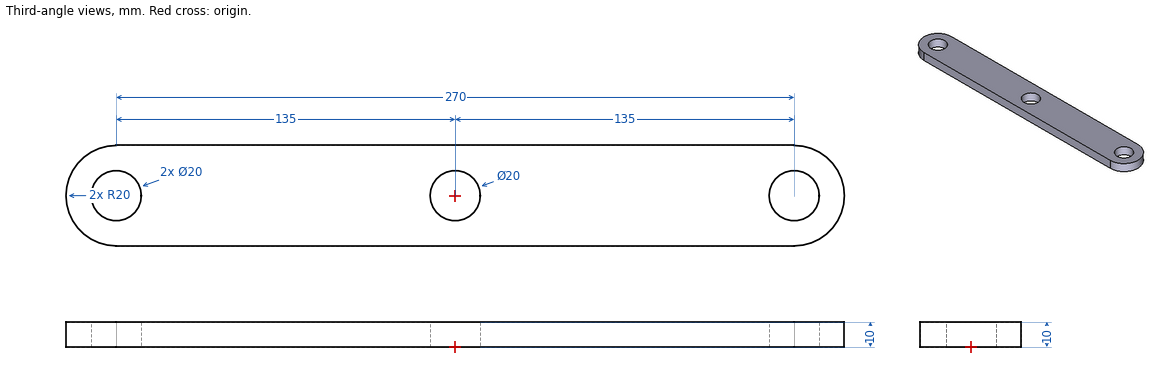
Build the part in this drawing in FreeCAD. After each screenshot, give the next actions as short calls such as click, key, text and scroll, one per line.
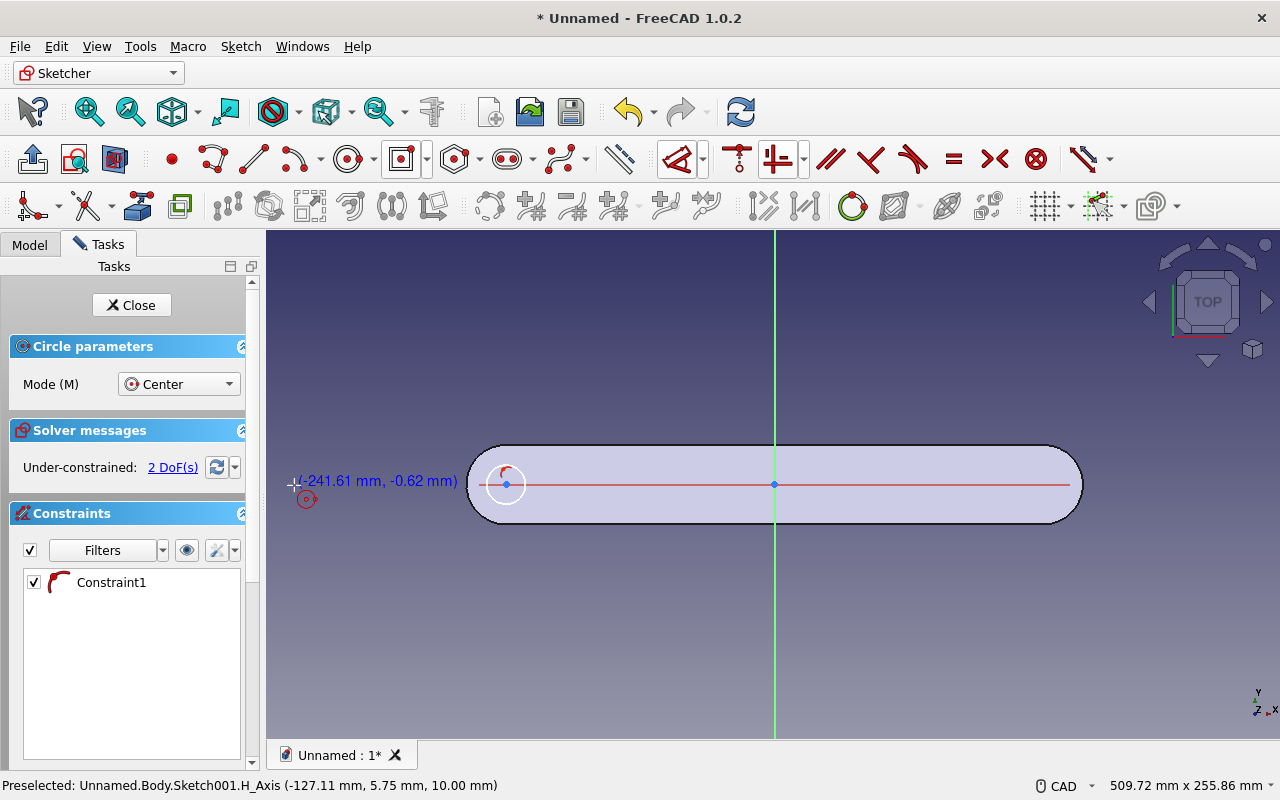
click(1043, 485)
click(1057, 471)
key(Escape)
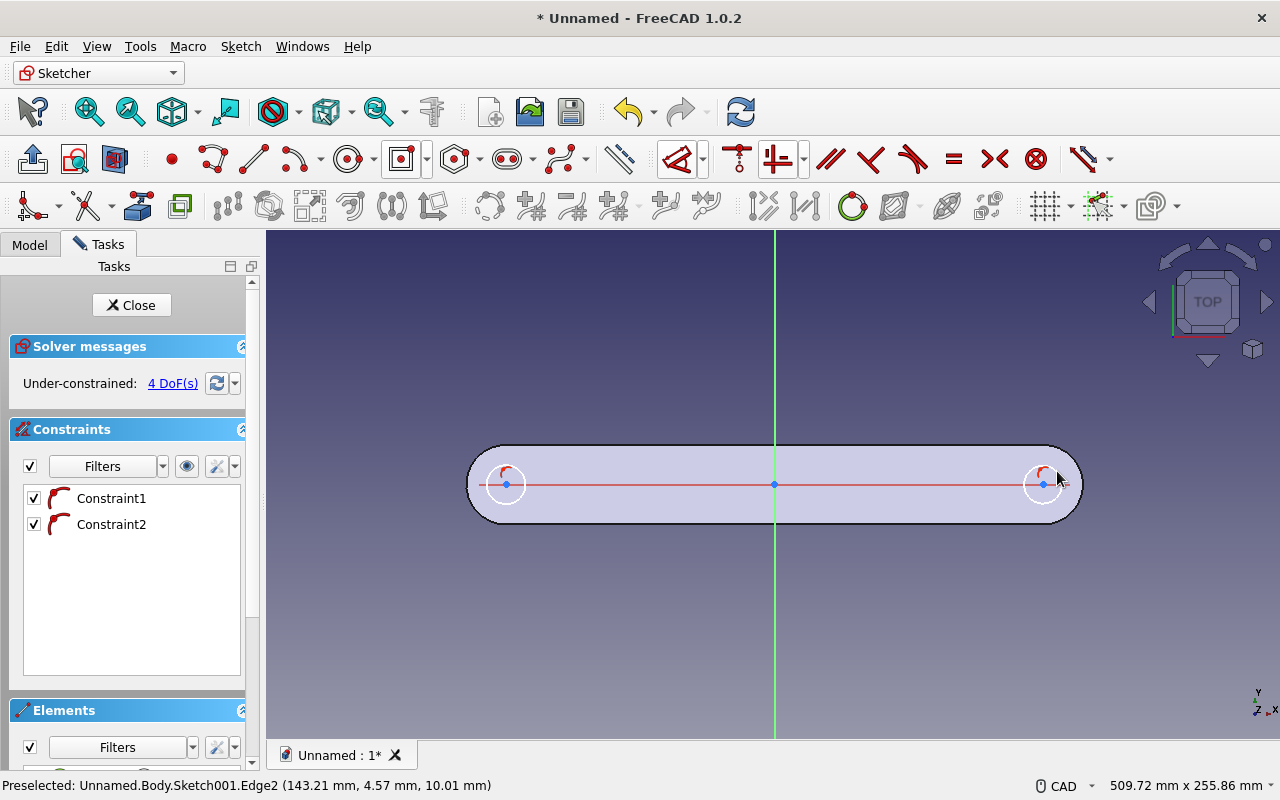
click(520, 471)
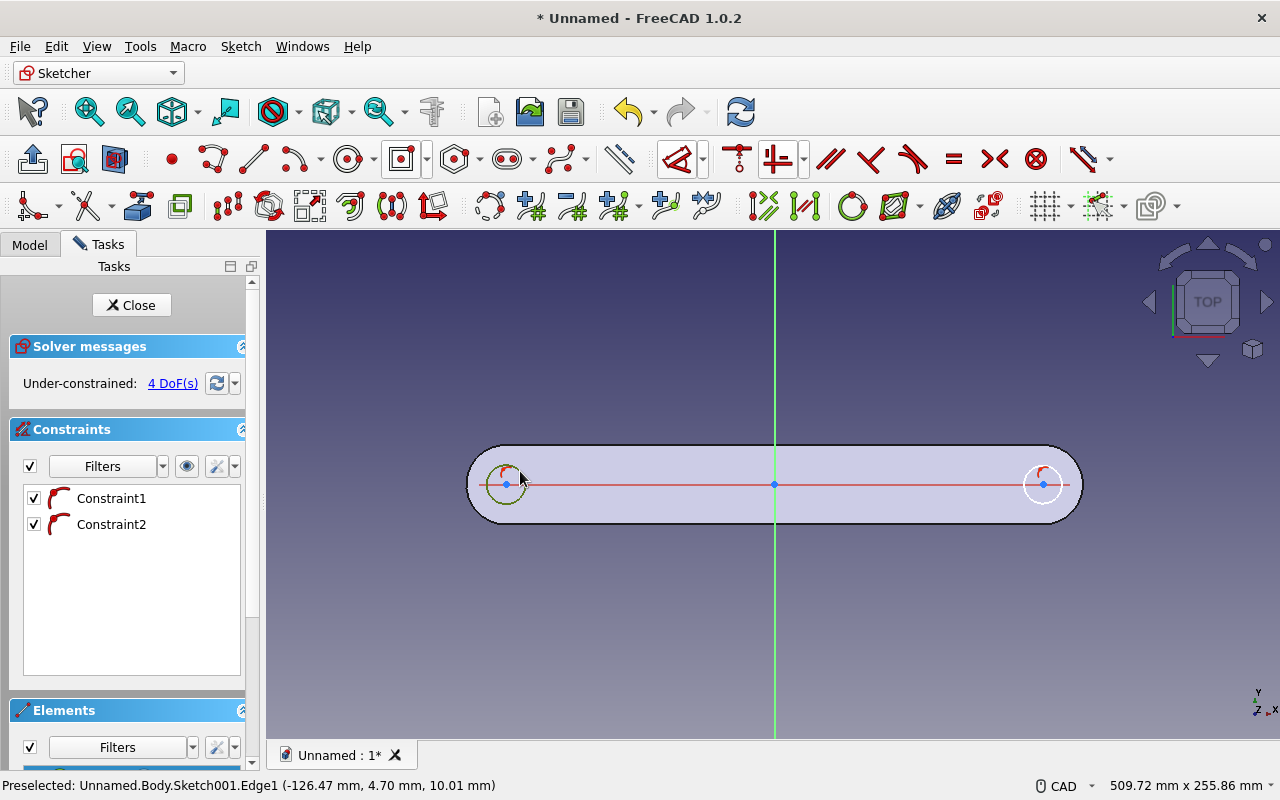
click(1056, 471)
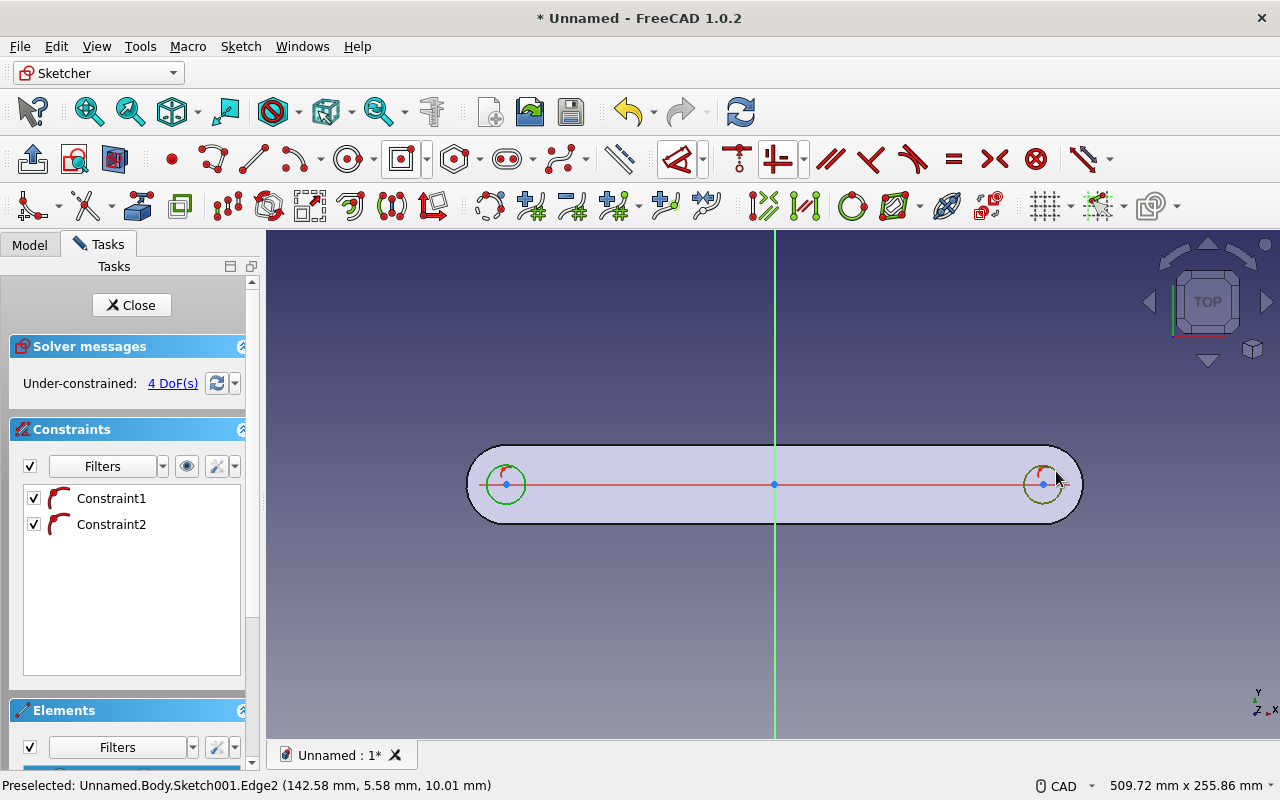
click(954, 160)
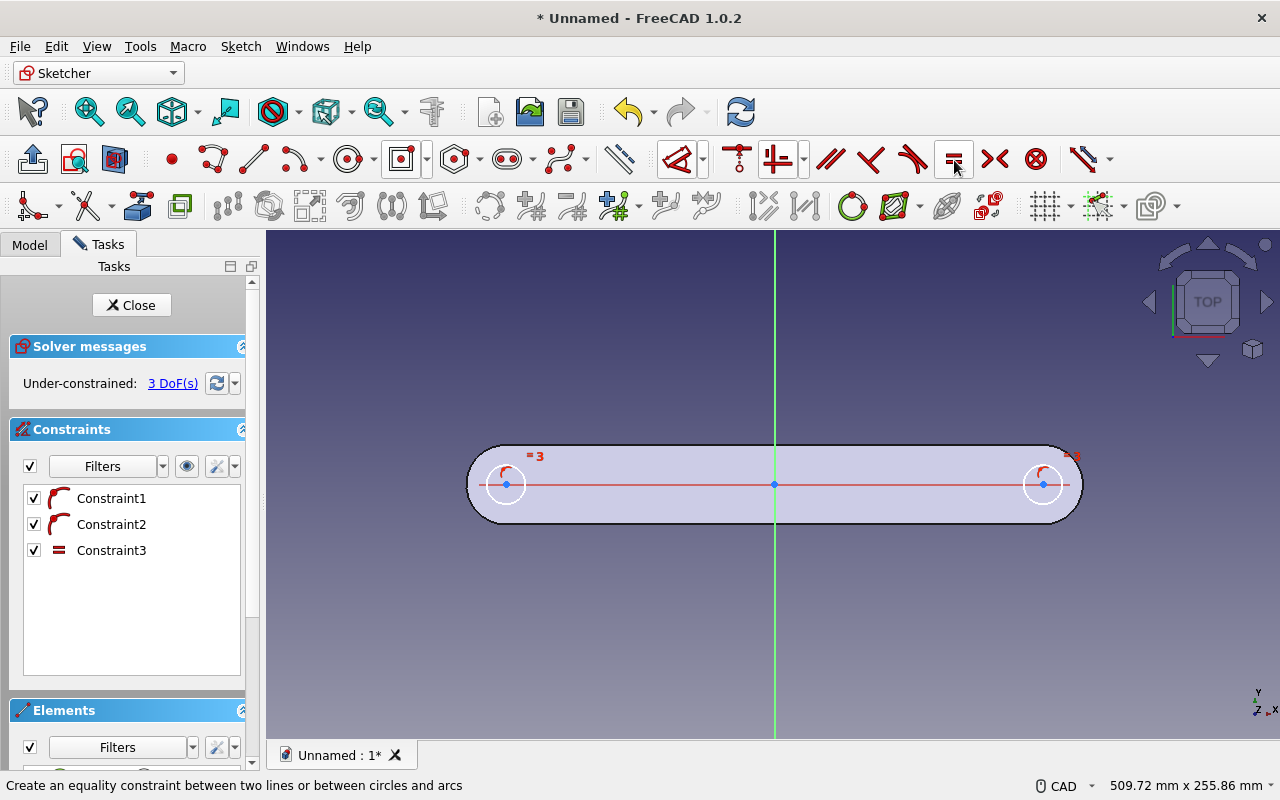
click(520, 471)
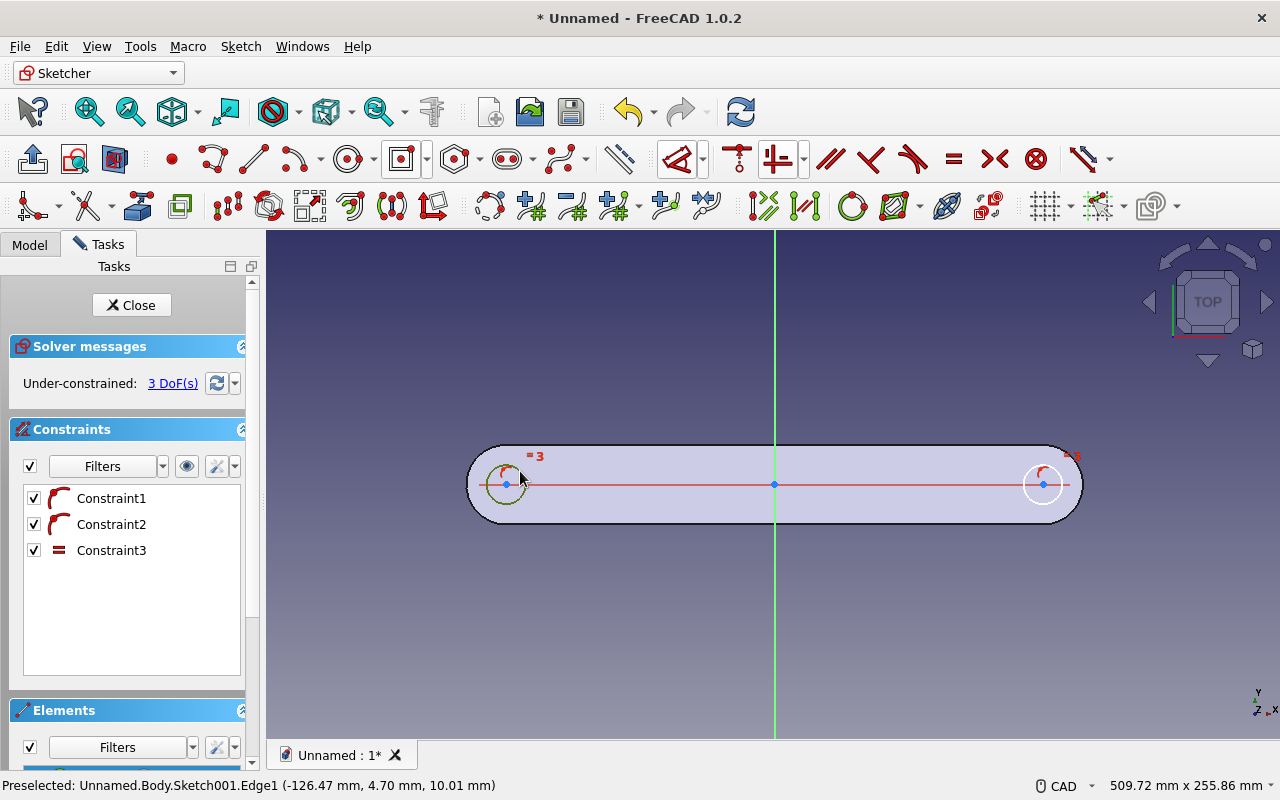
key(k)
key(o)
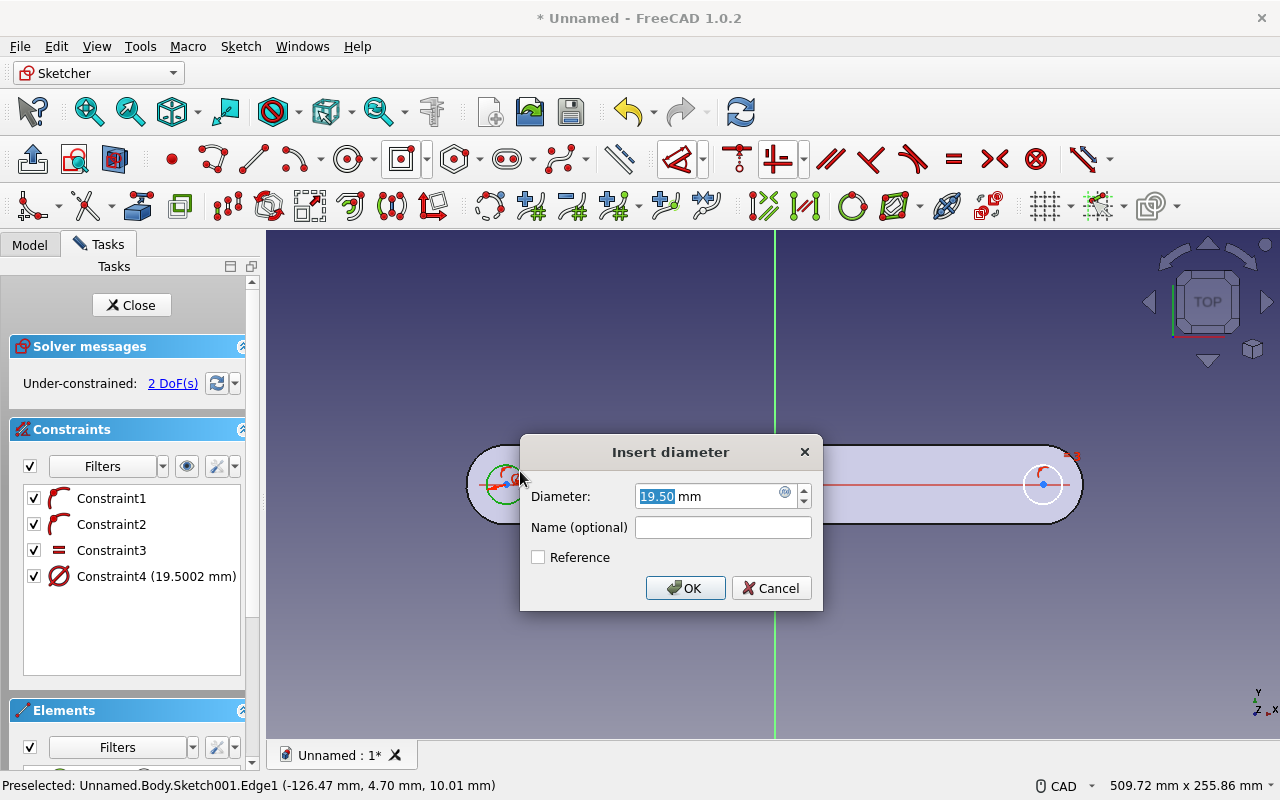
text(20)
key(Return)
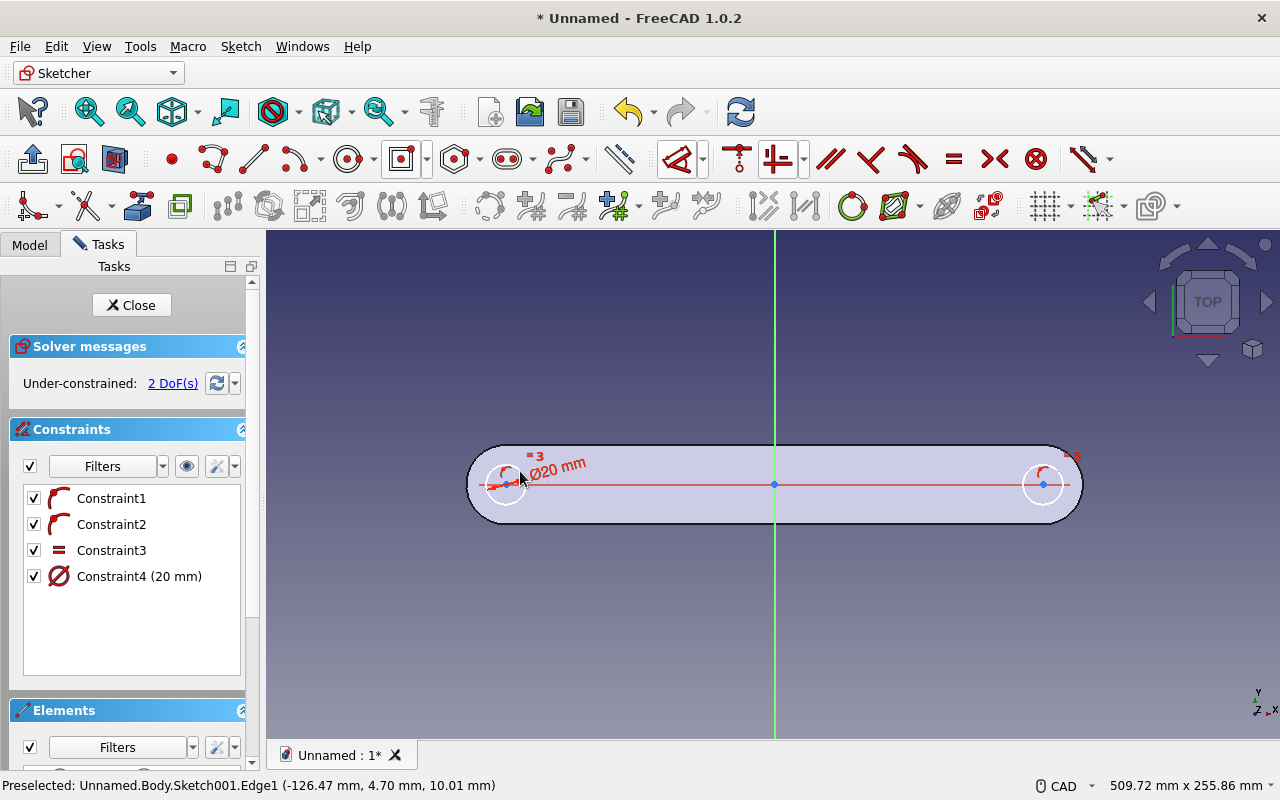
click(506, 485)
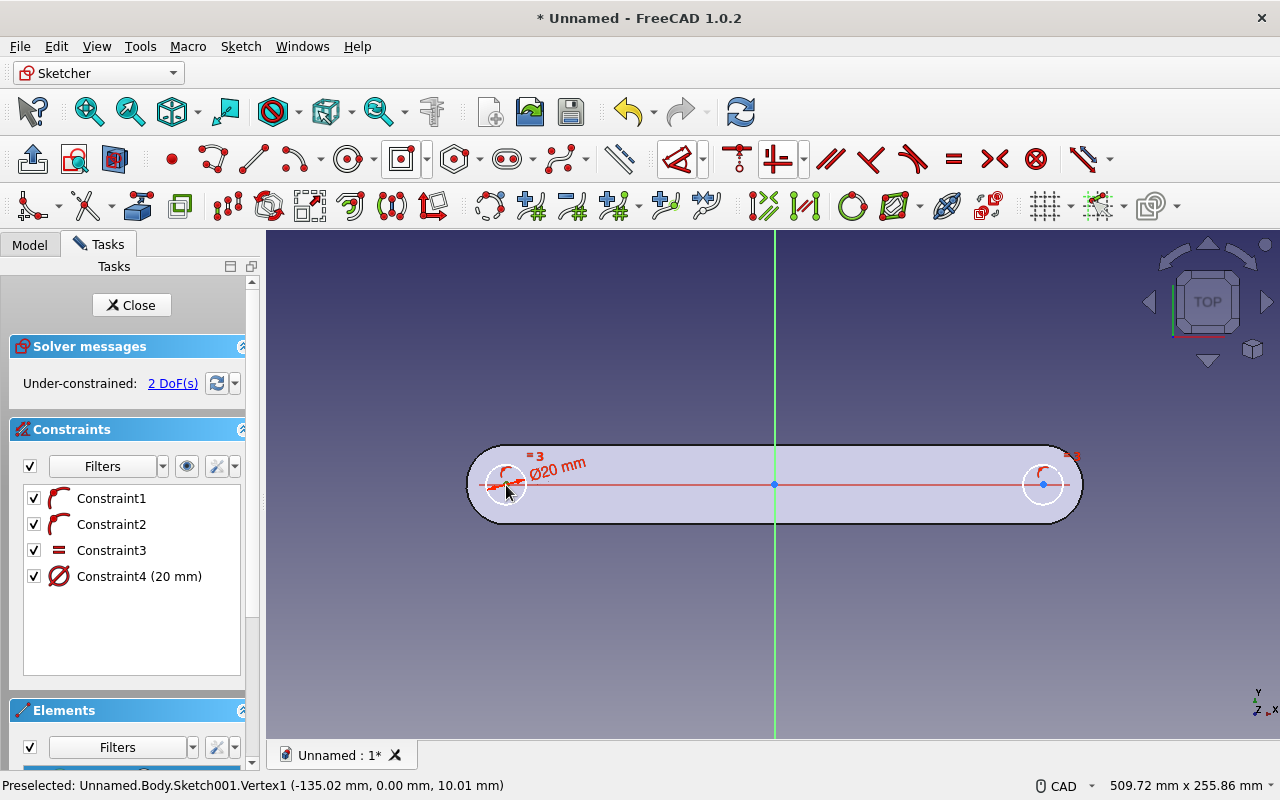
click(702, 160)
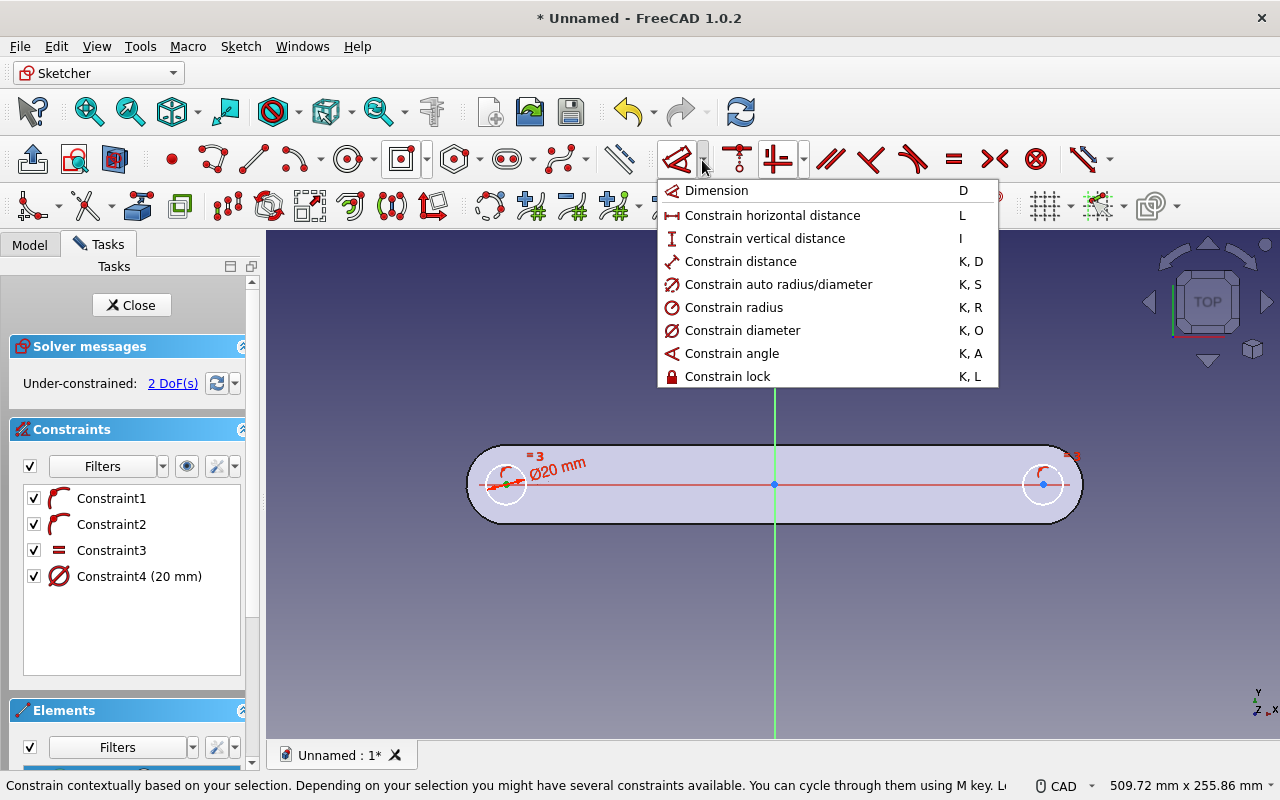
click(828, 216)